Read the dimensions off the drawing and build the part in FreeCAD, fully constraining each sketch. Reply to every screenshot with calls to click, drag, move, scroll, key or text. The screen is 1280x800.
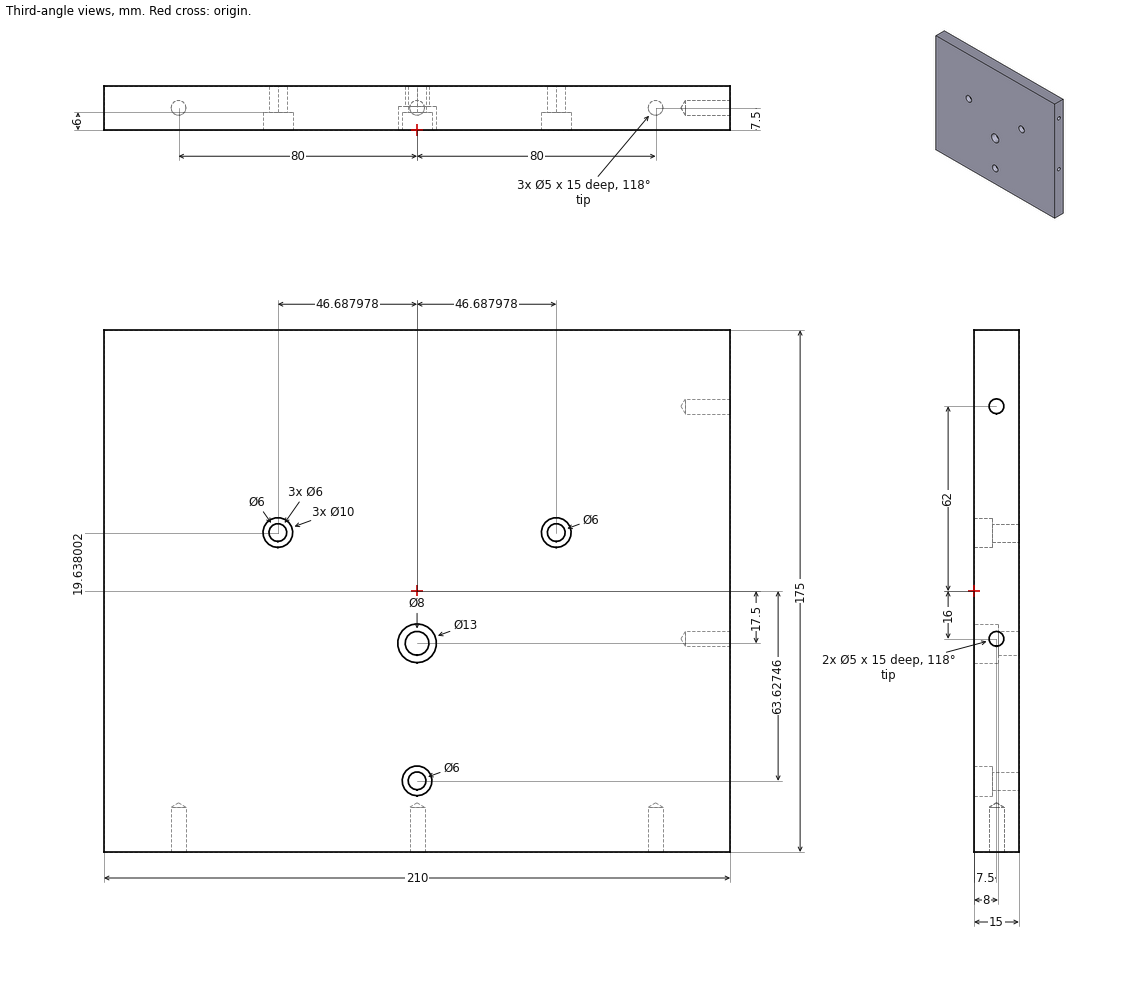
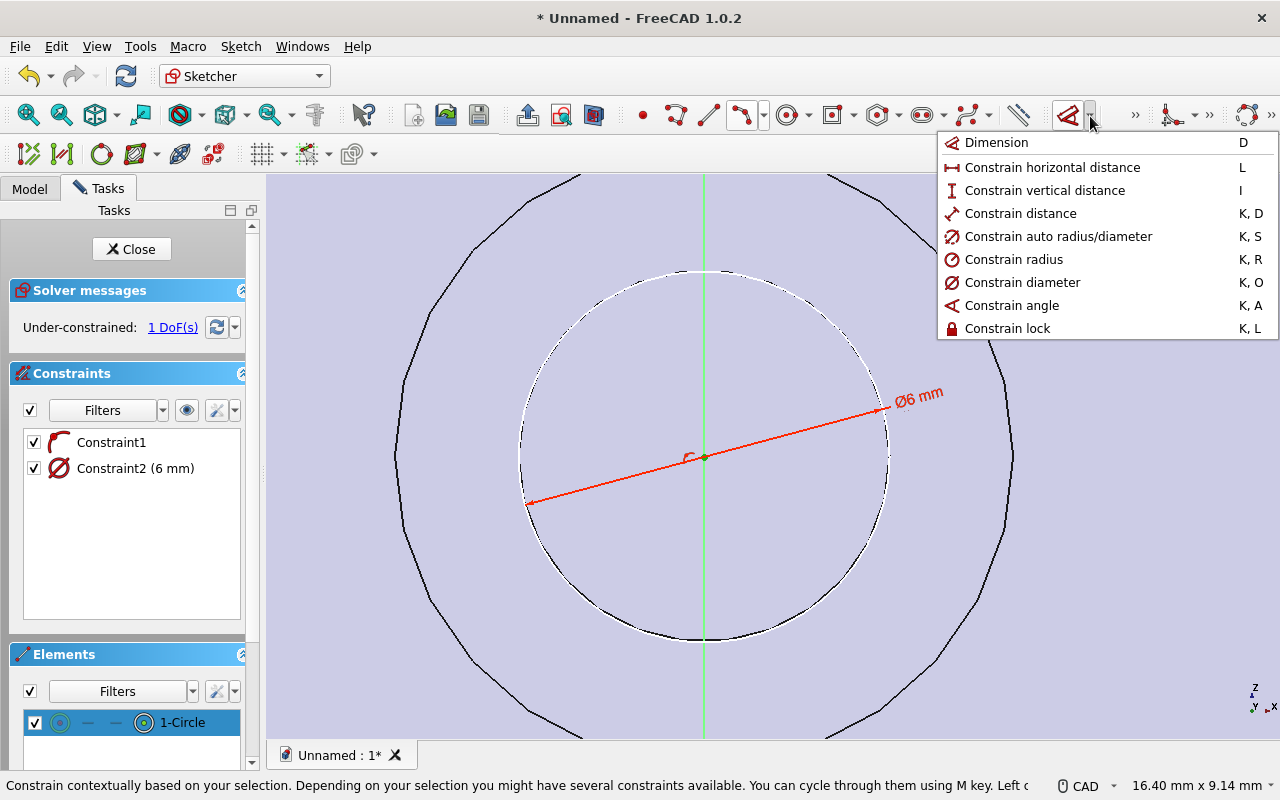
click(1108, 190)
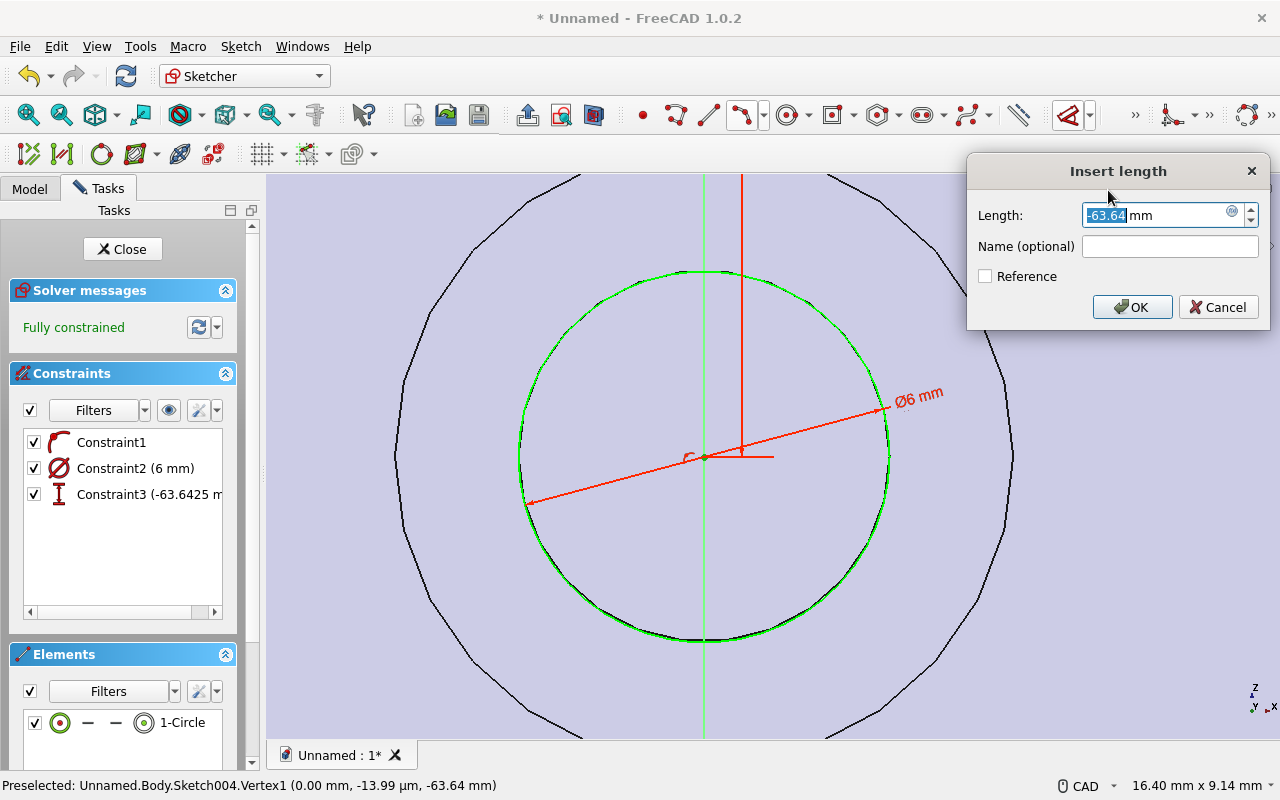
text(-63.62746)
key(Return)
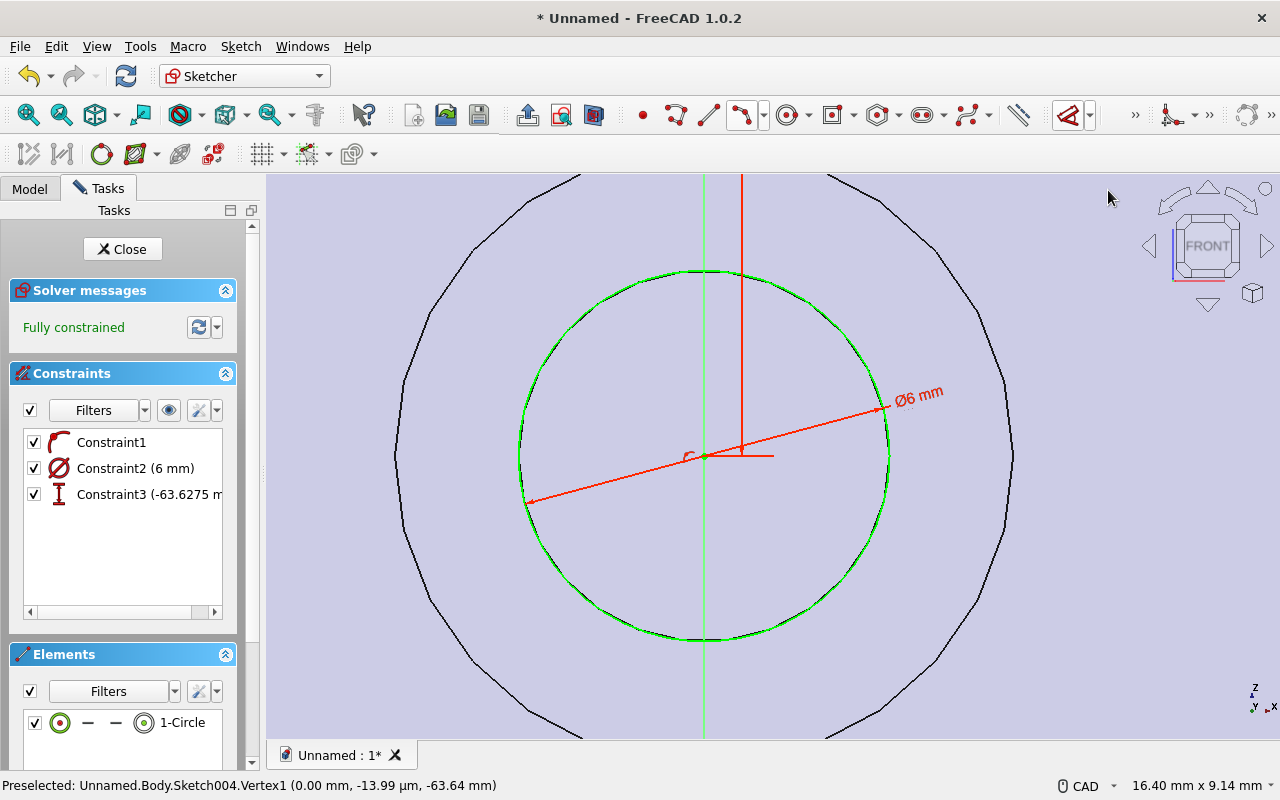
click(123, 249)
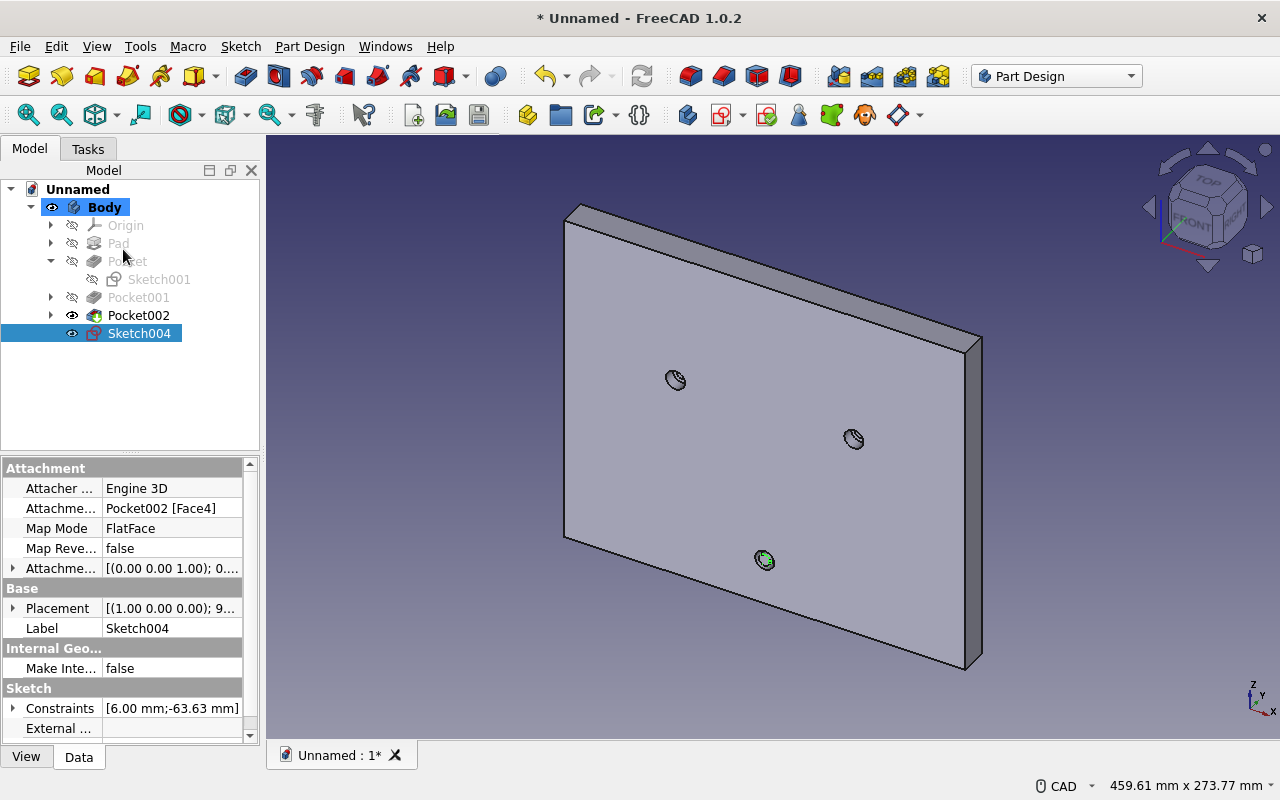
click(246, 76)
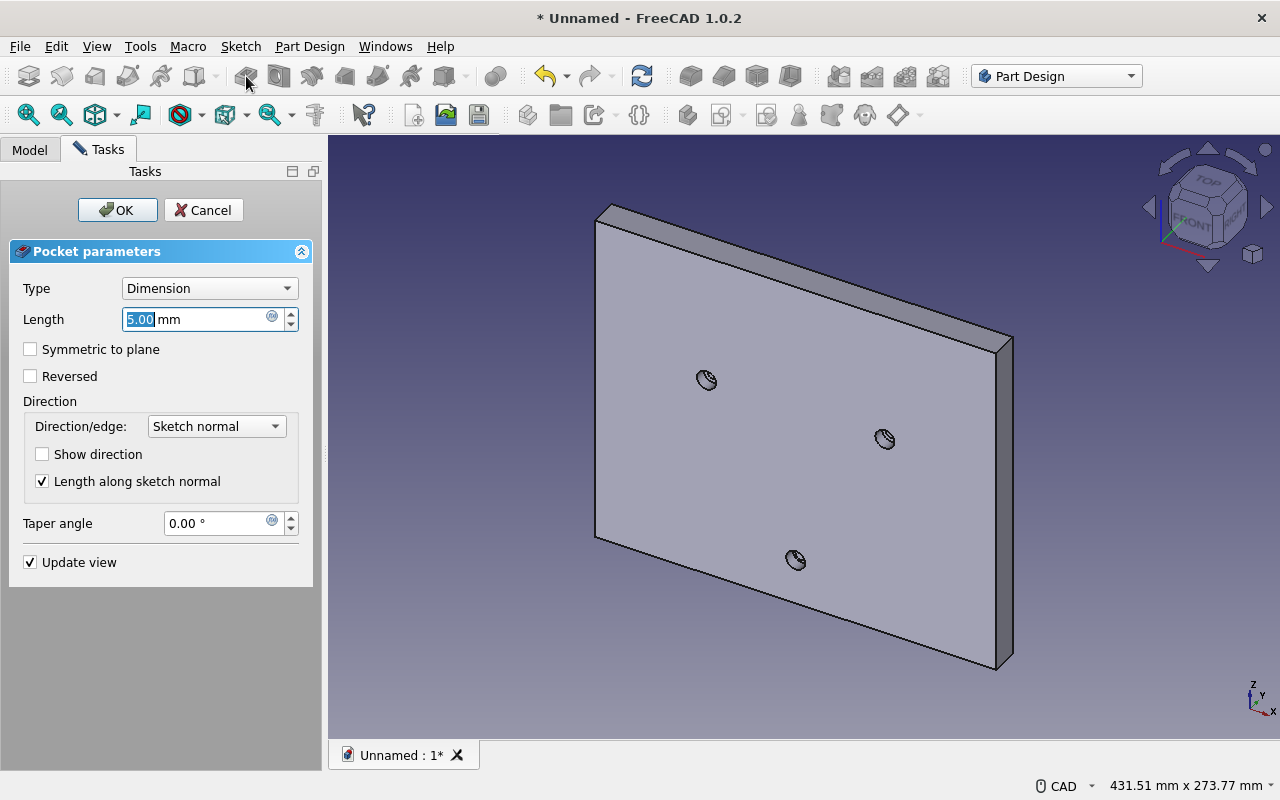
click(210, 288)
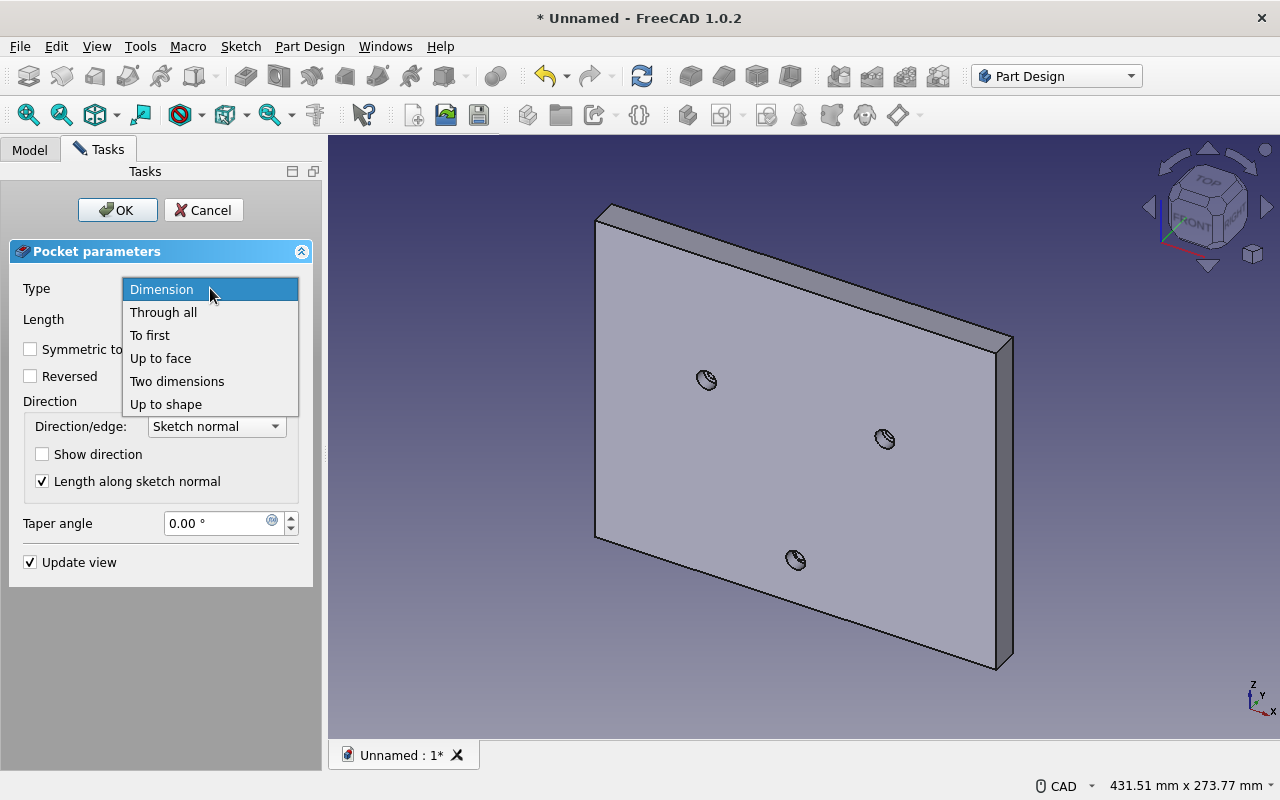
click(208, 336)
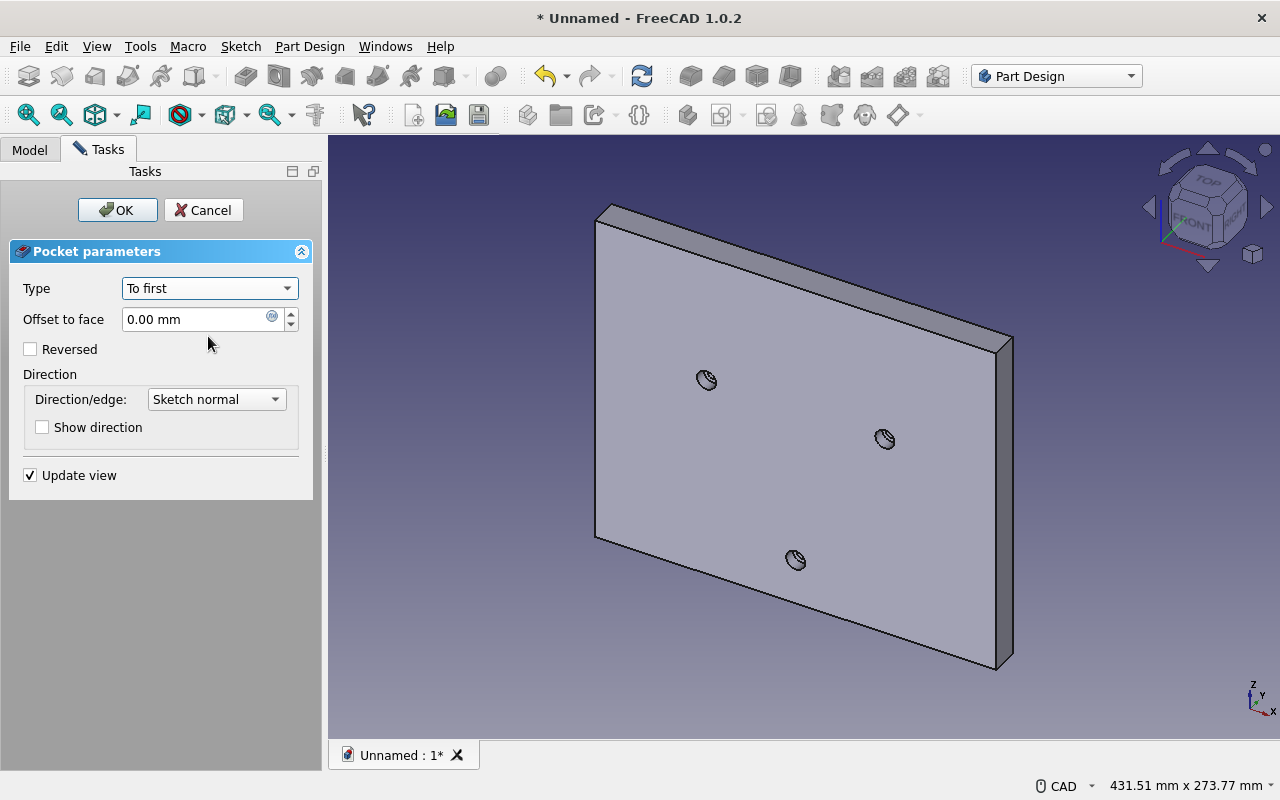
click(118, 210)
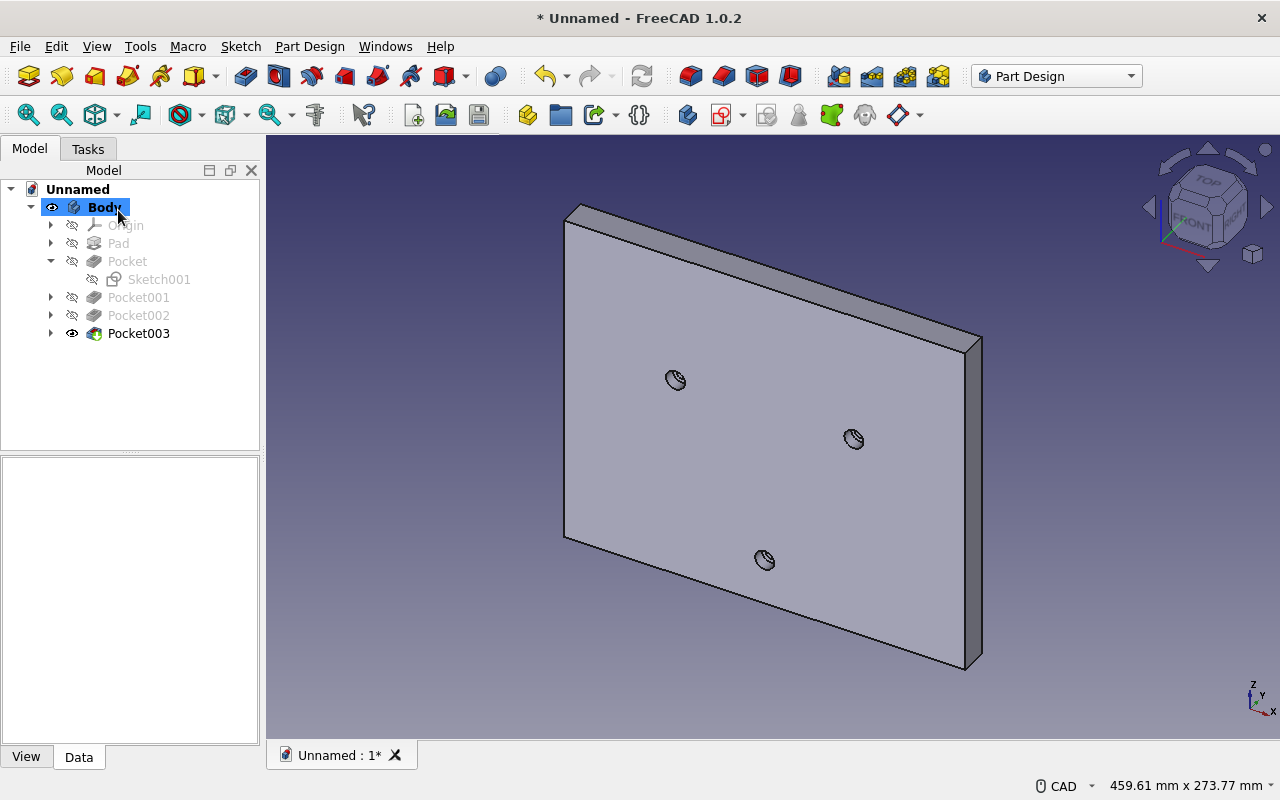
click(974, 457)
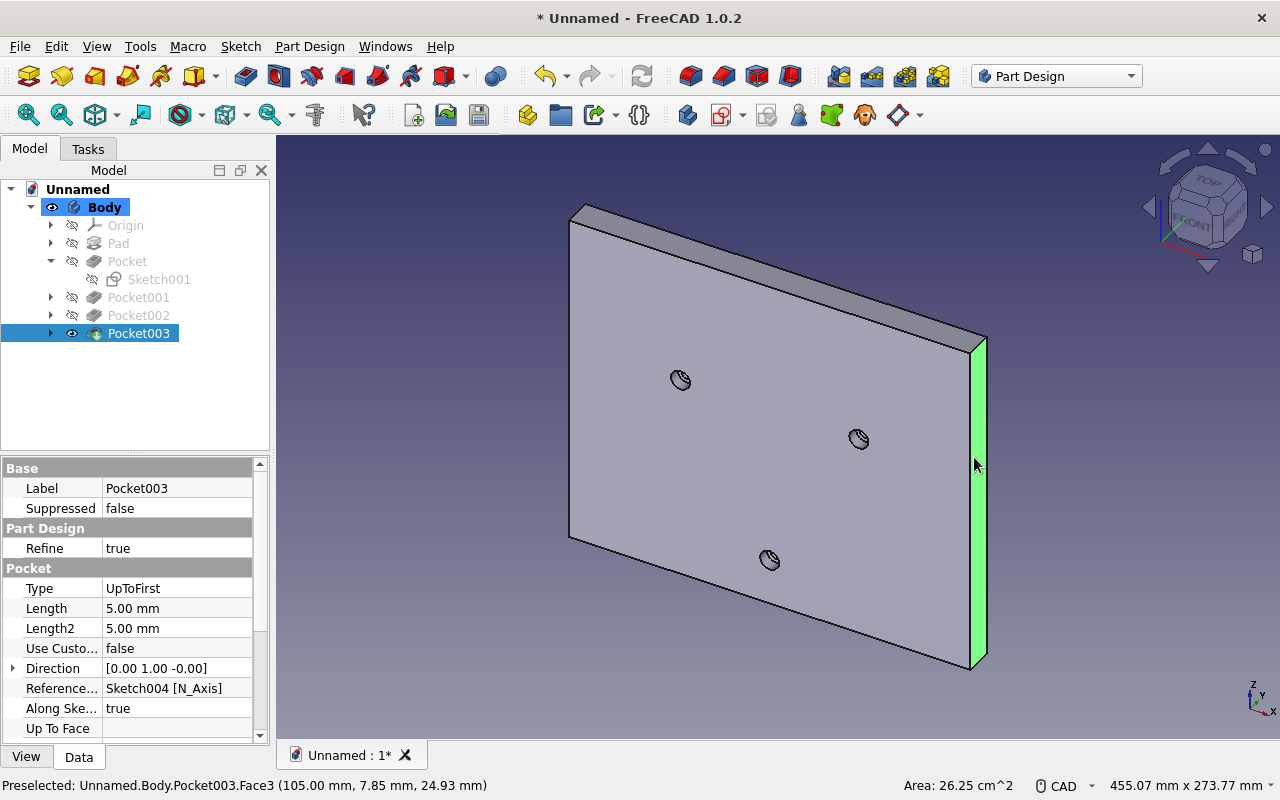
click(720, 116)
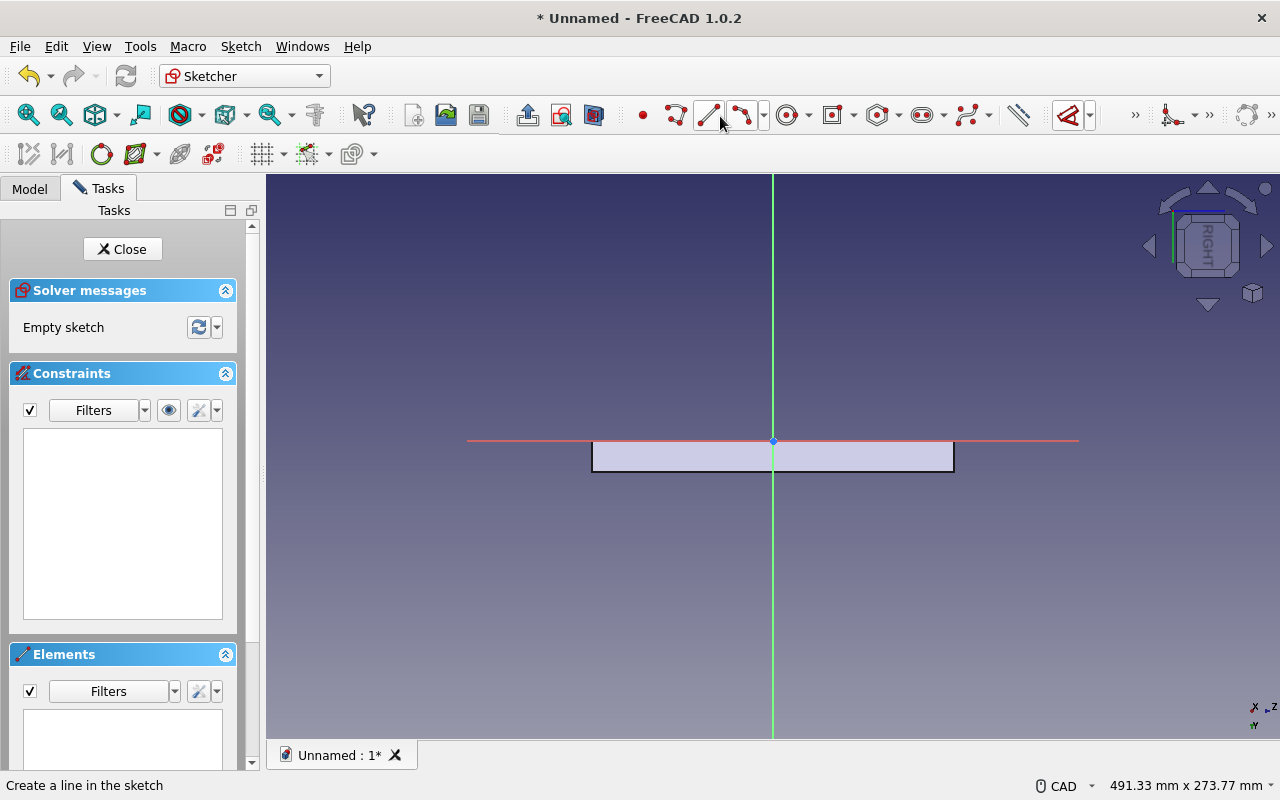
scroll(870, 449, up, 6)